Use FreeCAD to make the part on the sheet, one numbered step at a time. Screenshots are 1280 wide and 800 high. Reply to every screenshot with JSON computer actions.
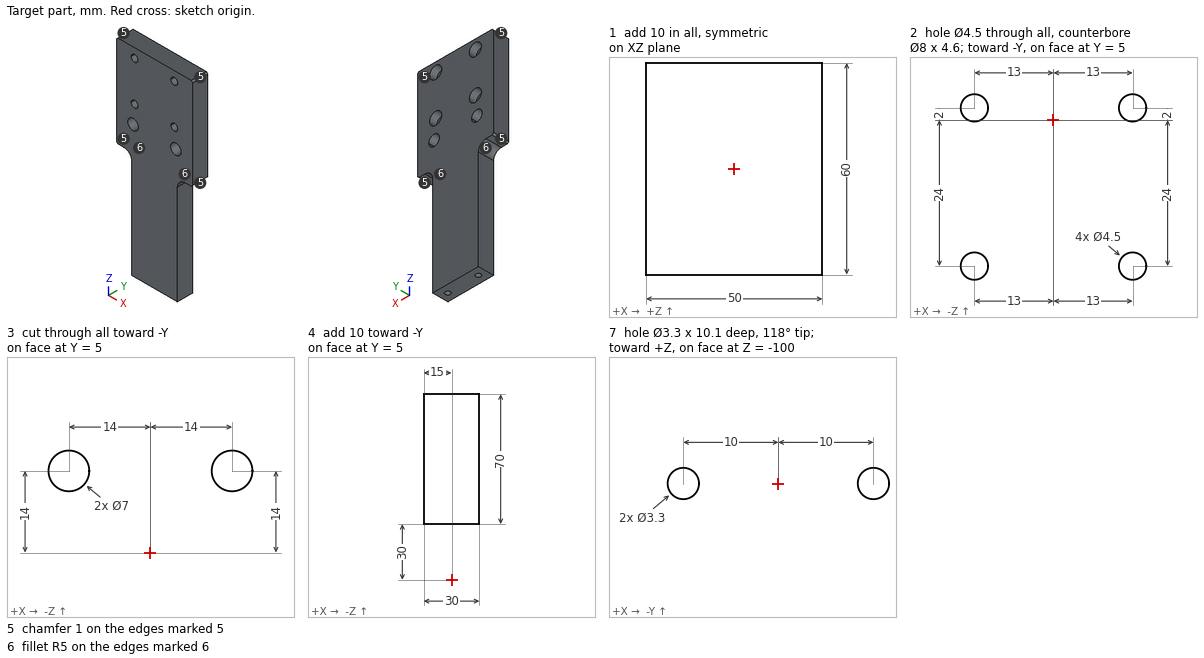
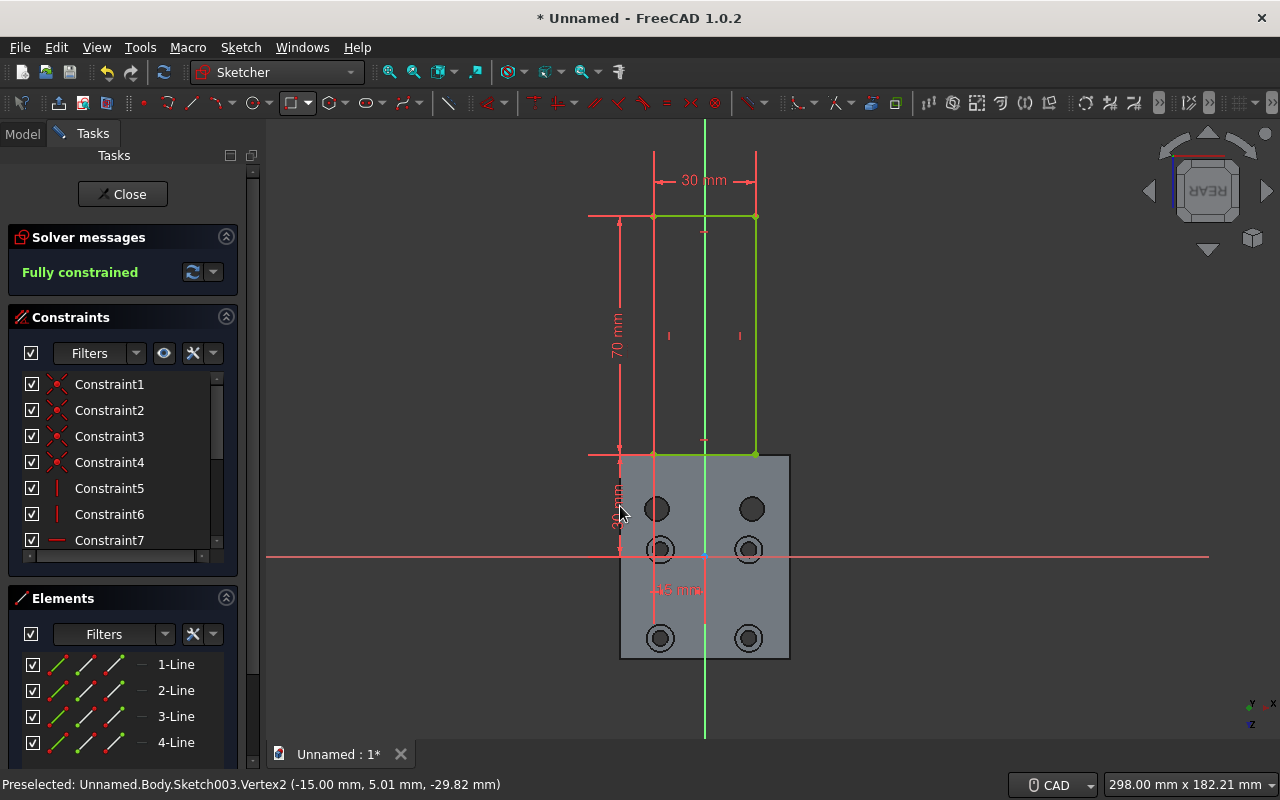
{"action": "left_click", "coordinate": [123, 194]}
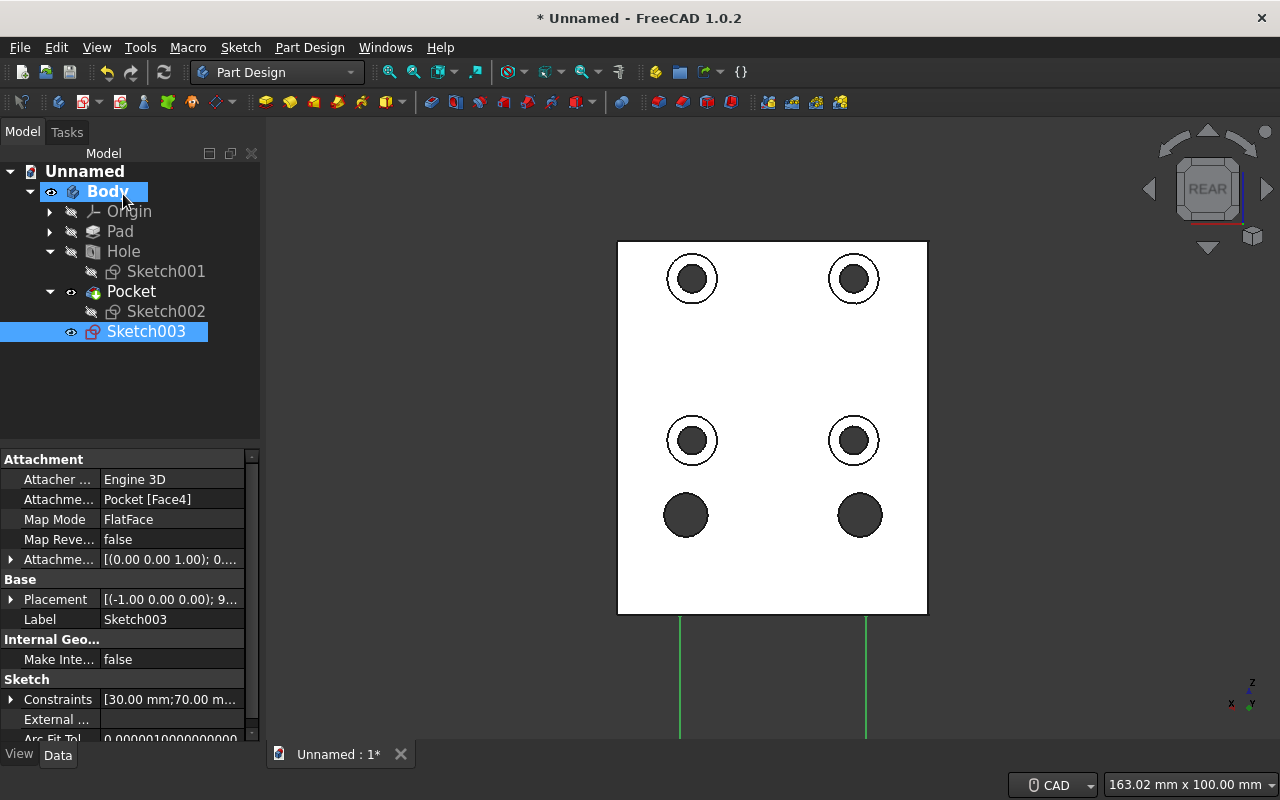
{"action": "left_click", "coordinate": [266, 102]}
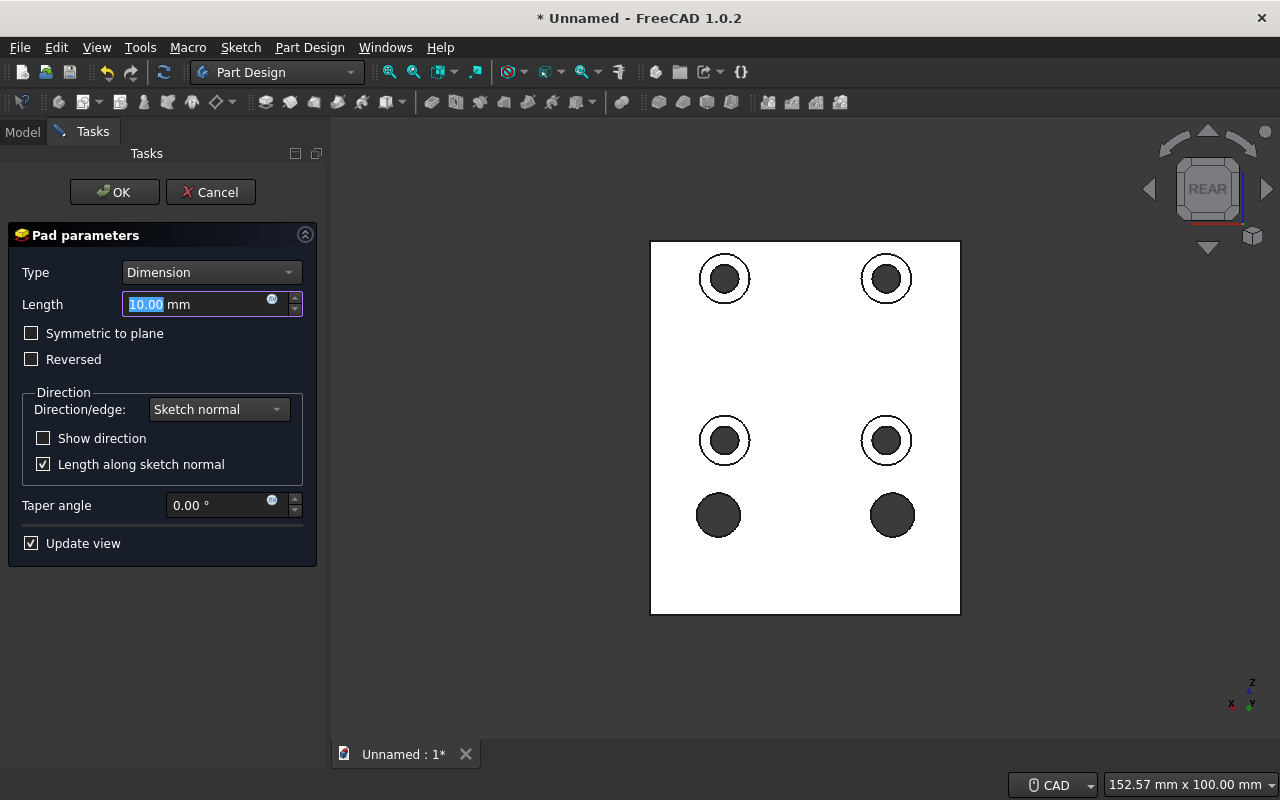
{"action": "type", "text": "10"}
{"action": "key", "text": "Tab"}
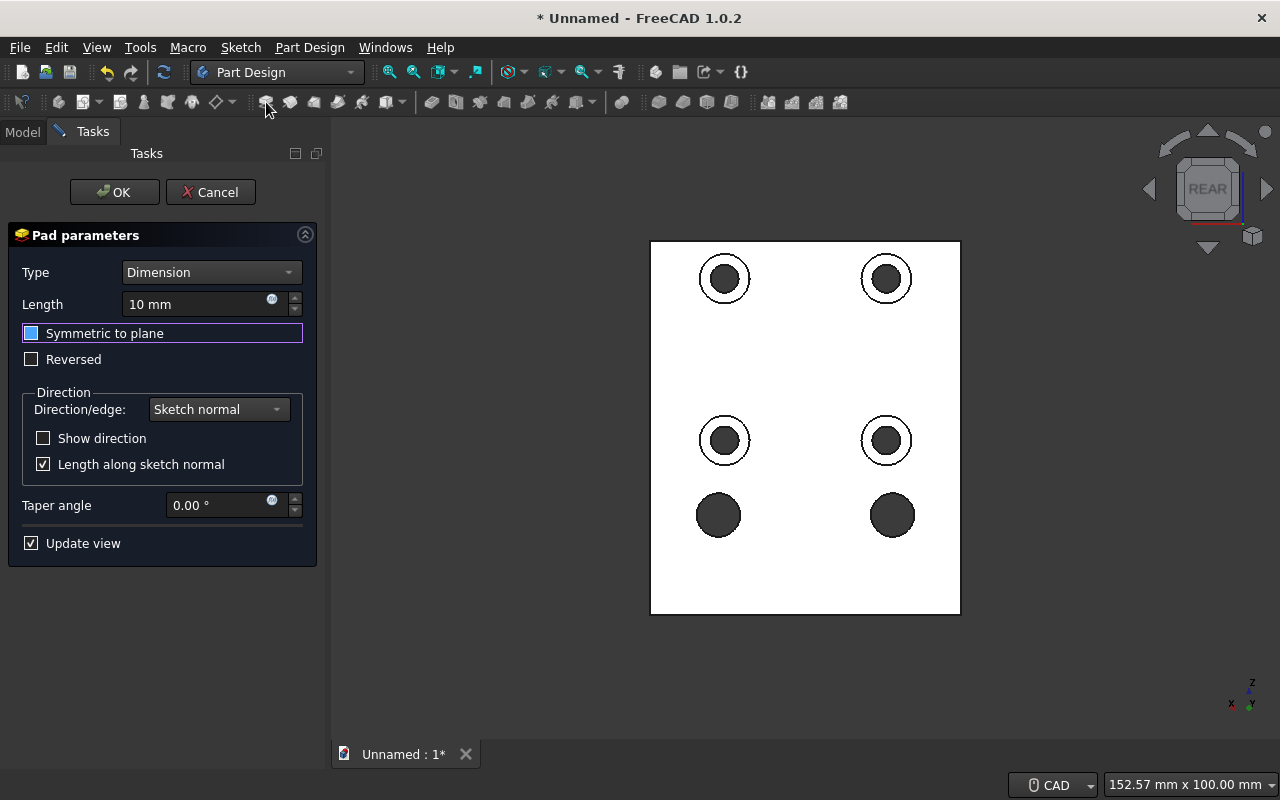
{"action": "left_click", "coordinate": [30, 359]}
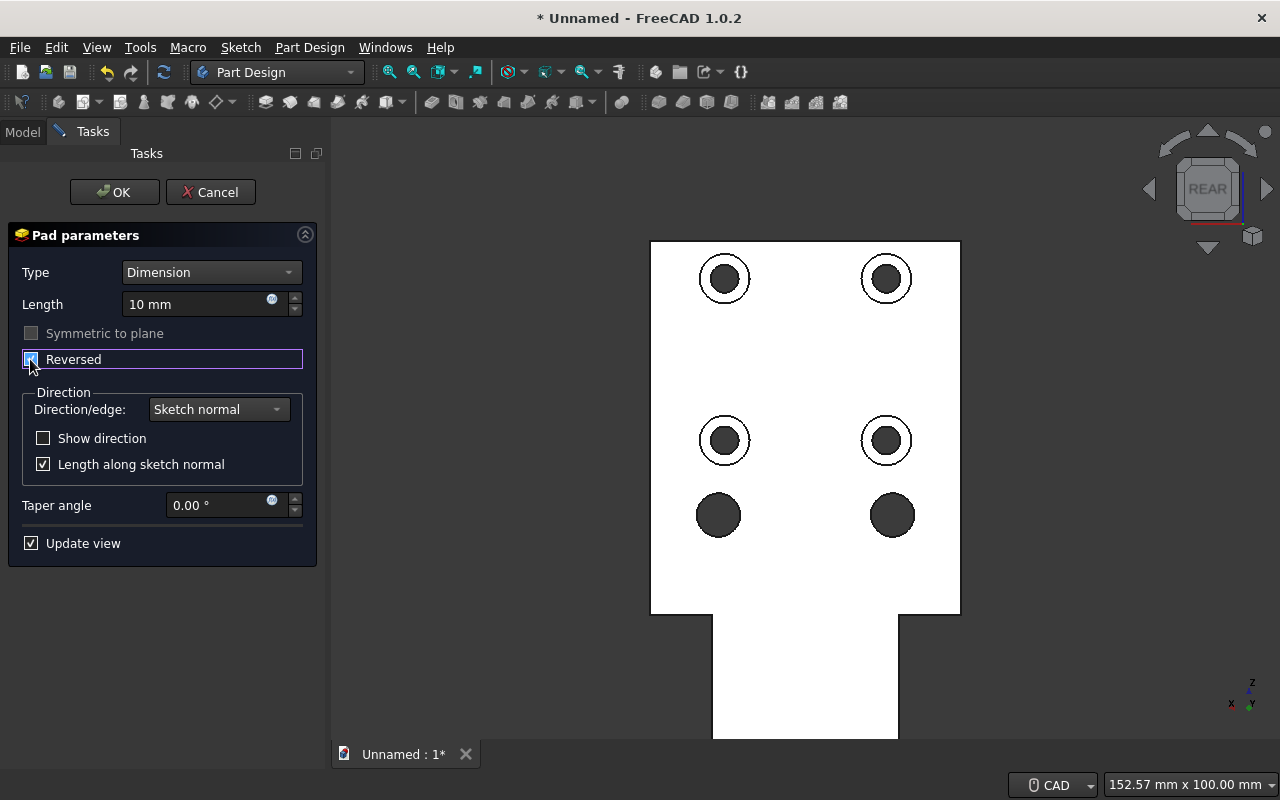
{"action": "left_click", "coordinate": [115, 192]}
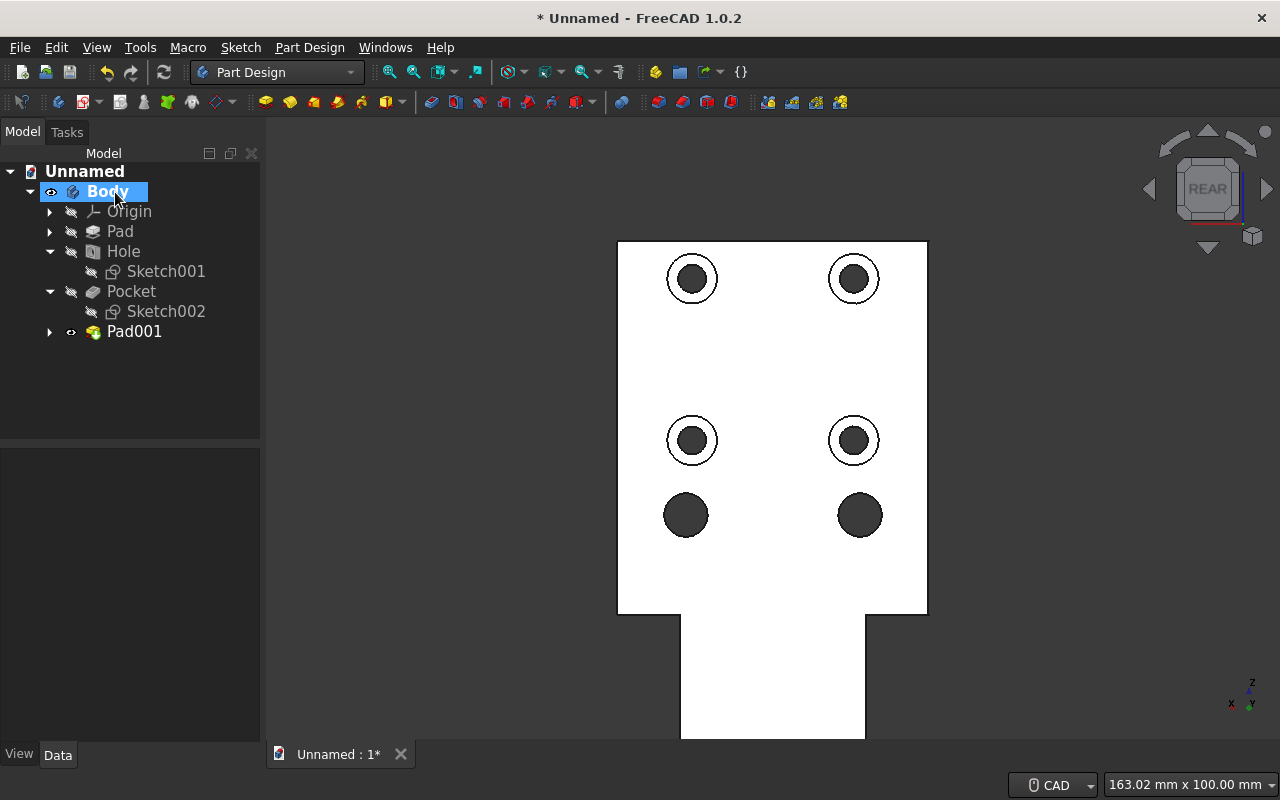
{"action": "left_click", "coordinate": [390, 72]}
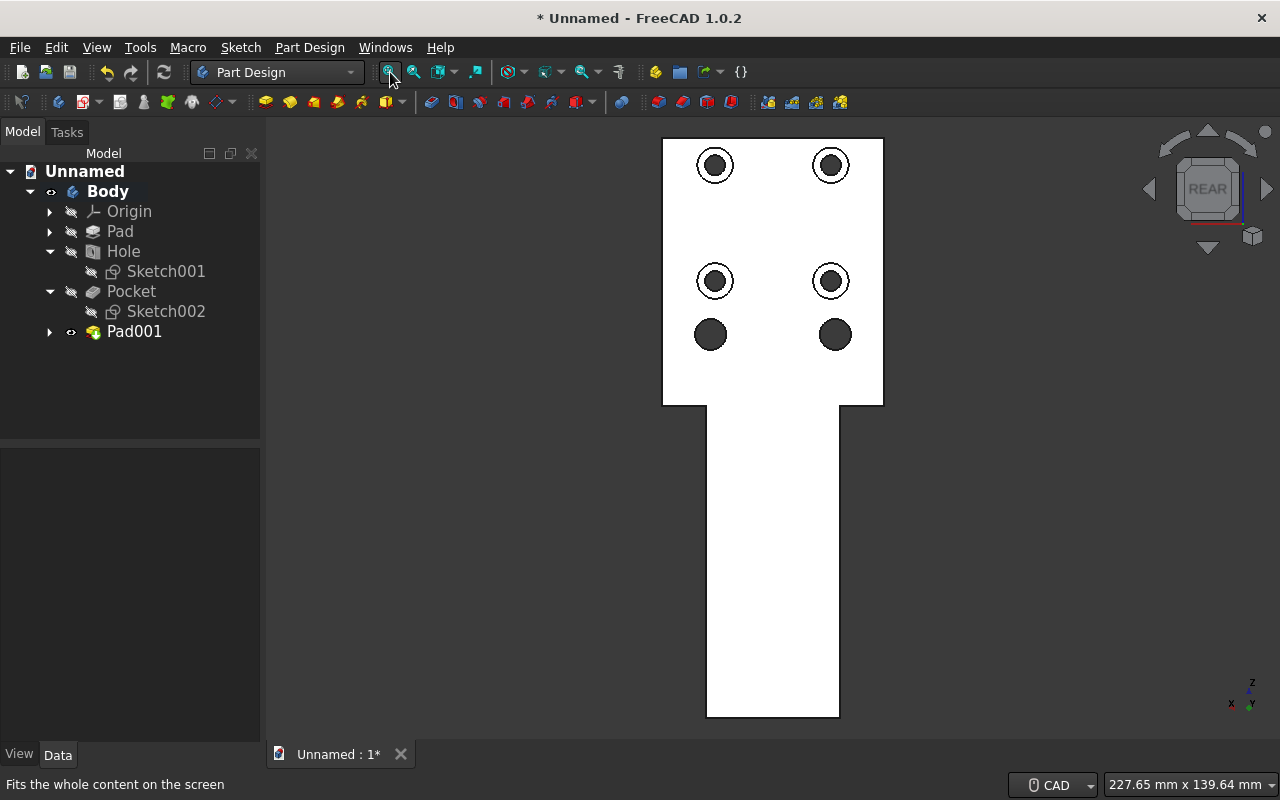
{"action": "key", "text": "0"}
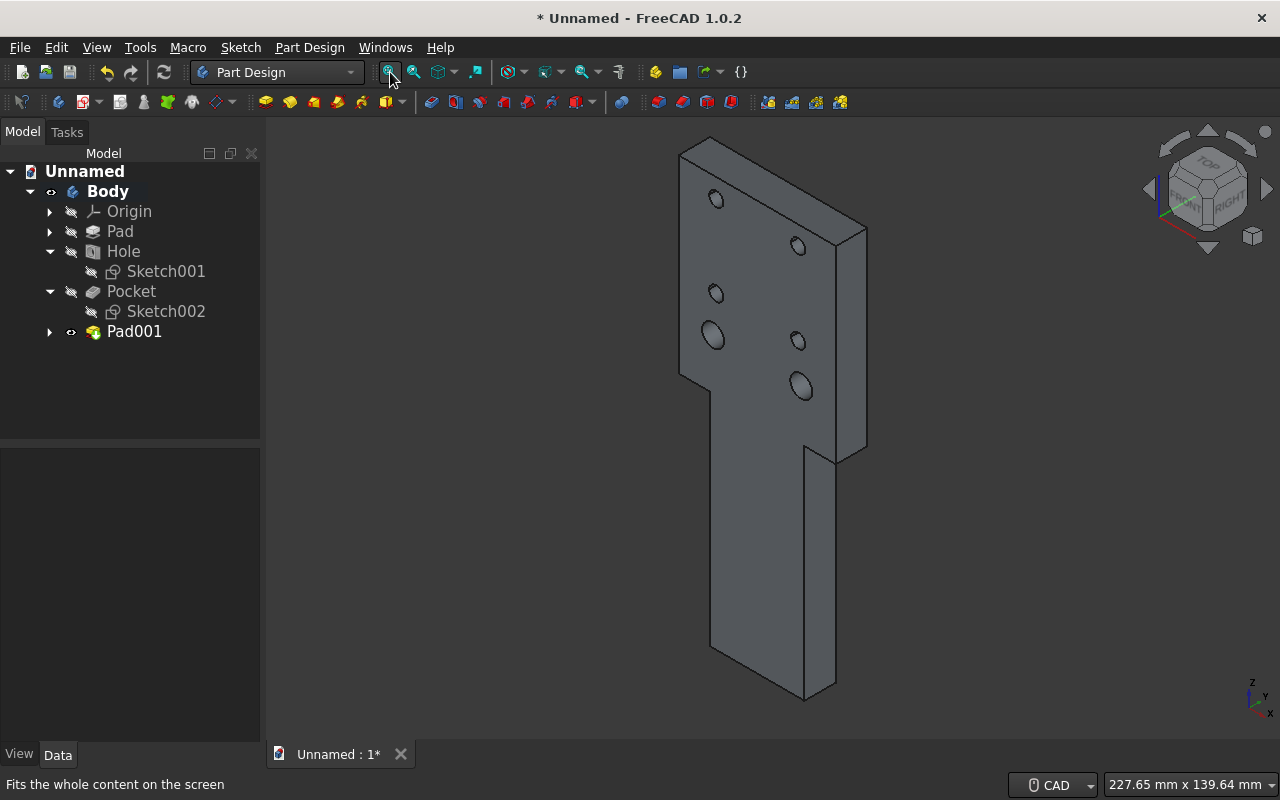
{"action": "left_click", "coordinate": [852, 236]}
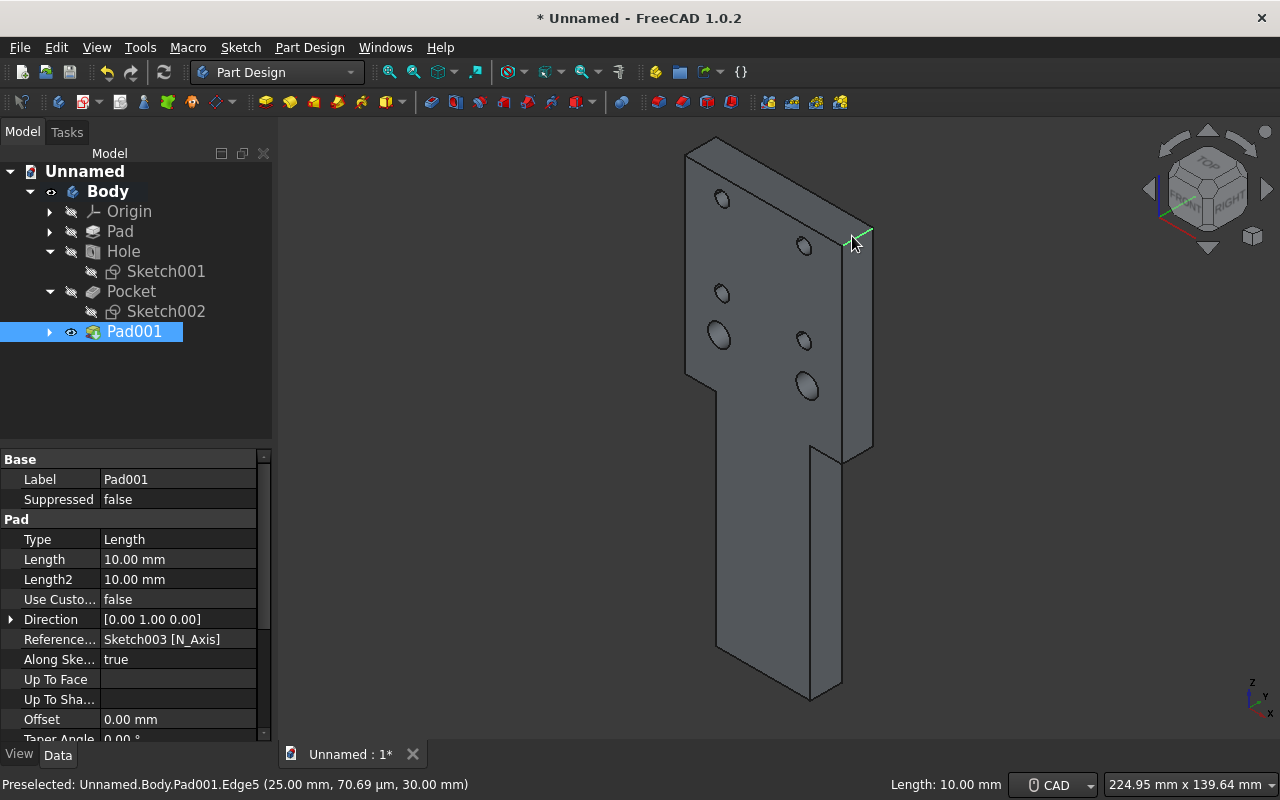
{"action": "key", "text": "2"}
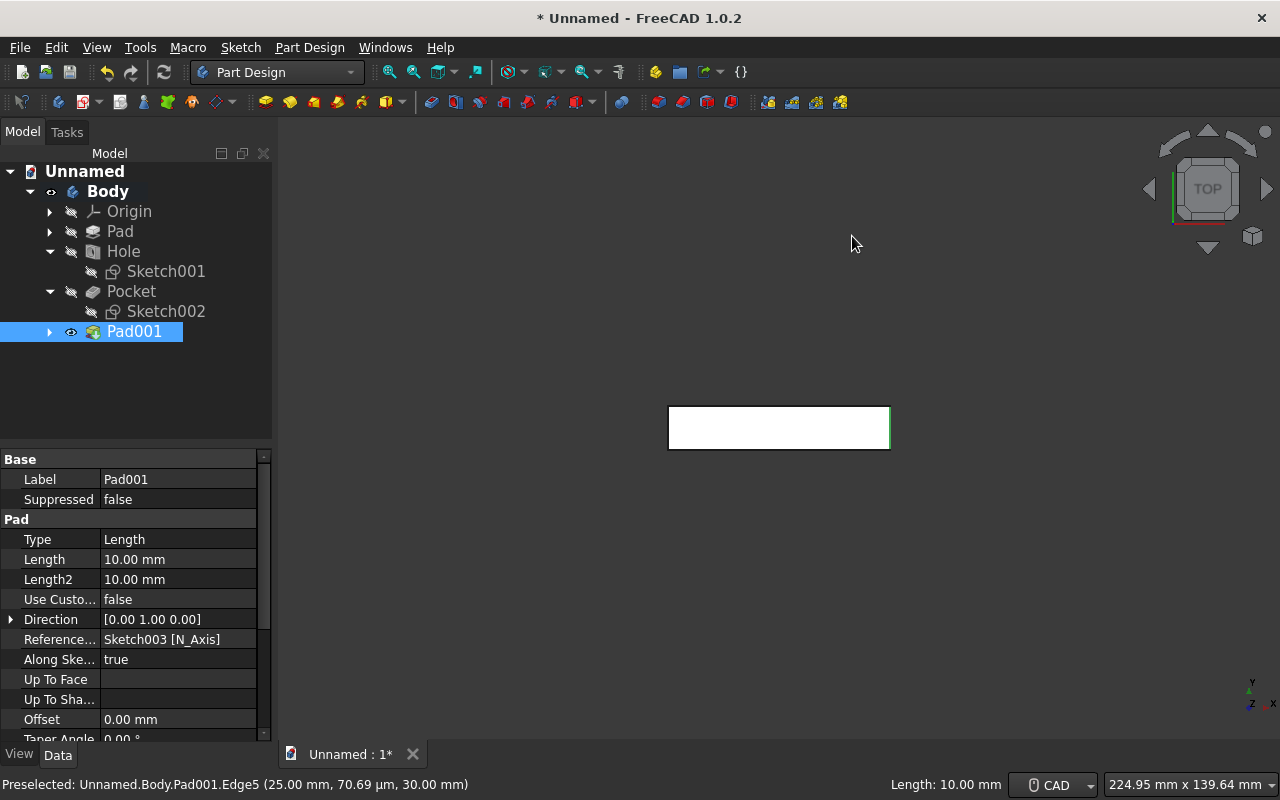
{"action": "left_click", "coordinate": [390, 72]}